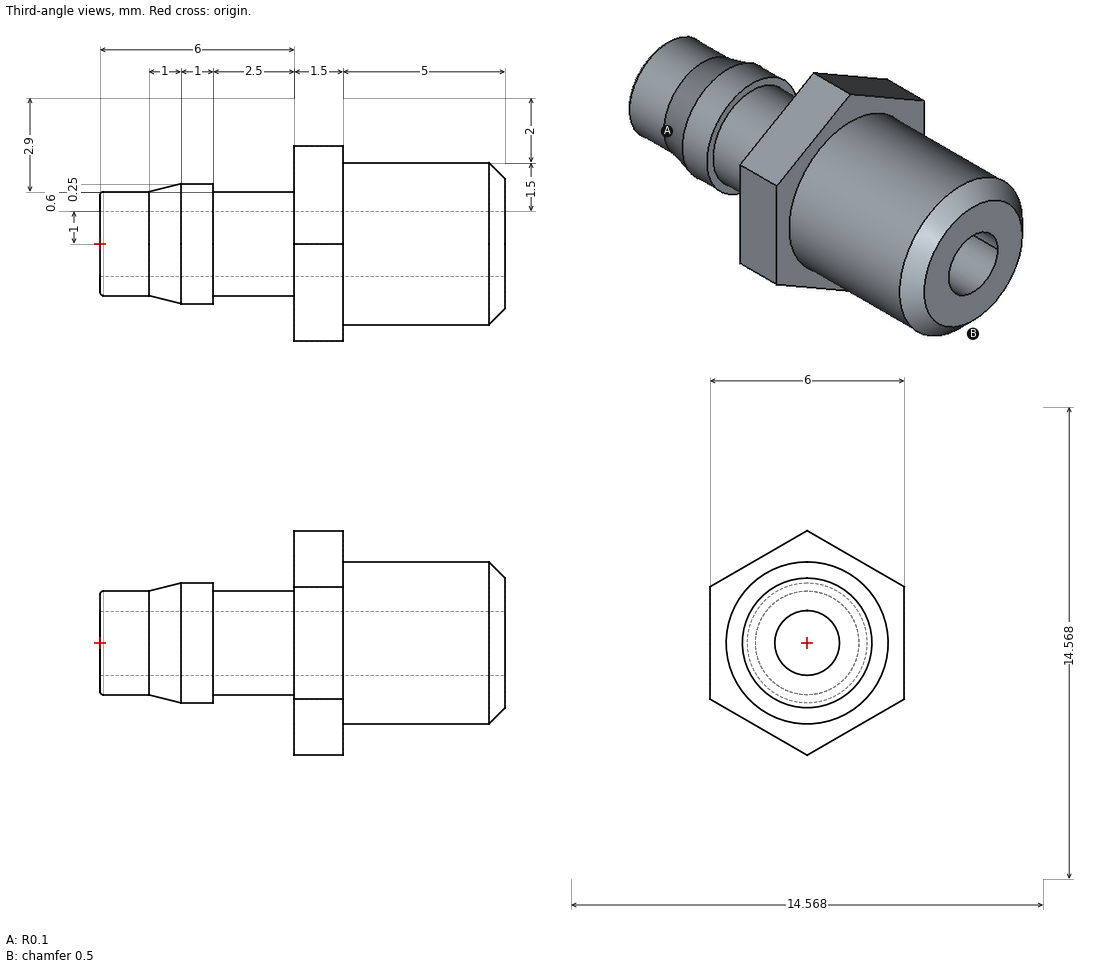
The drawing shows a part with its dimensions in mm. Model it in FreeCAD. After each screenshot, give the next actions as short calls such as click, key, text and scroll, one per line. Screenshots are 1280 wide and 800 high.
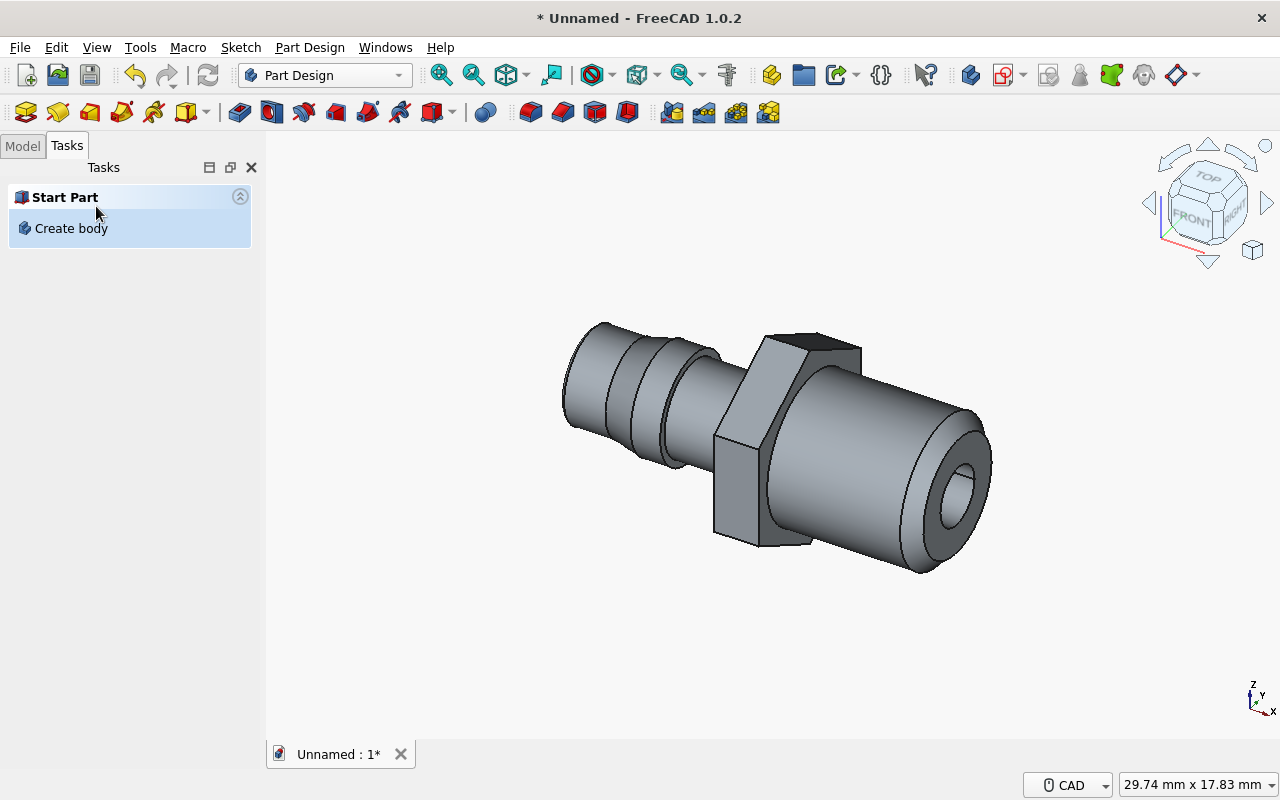
key(0)